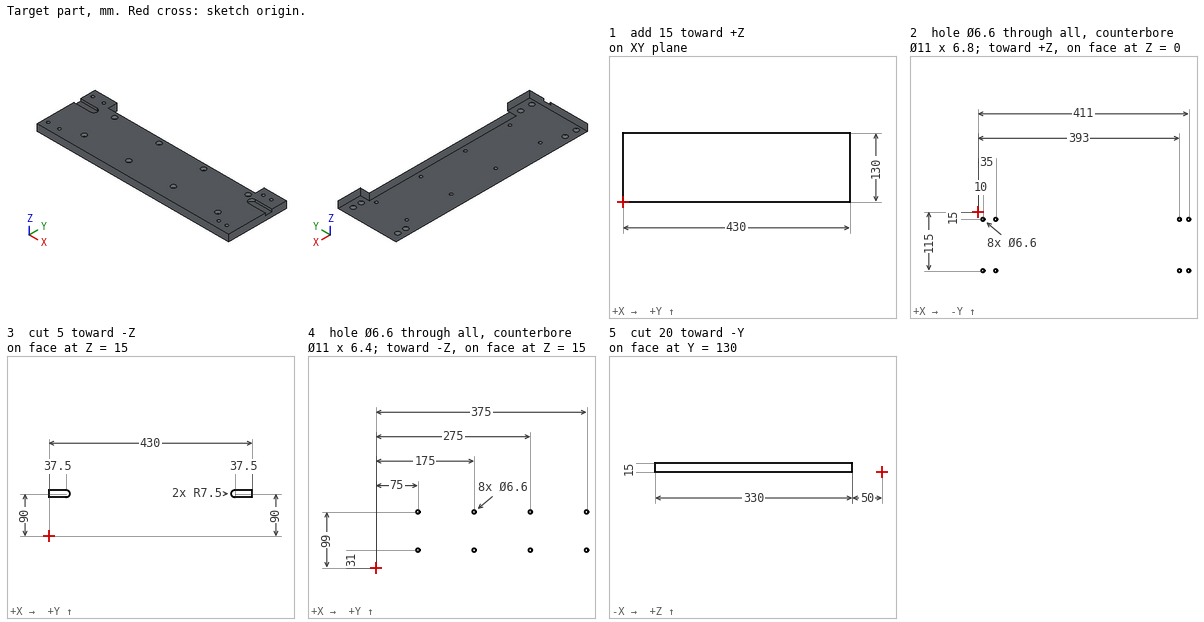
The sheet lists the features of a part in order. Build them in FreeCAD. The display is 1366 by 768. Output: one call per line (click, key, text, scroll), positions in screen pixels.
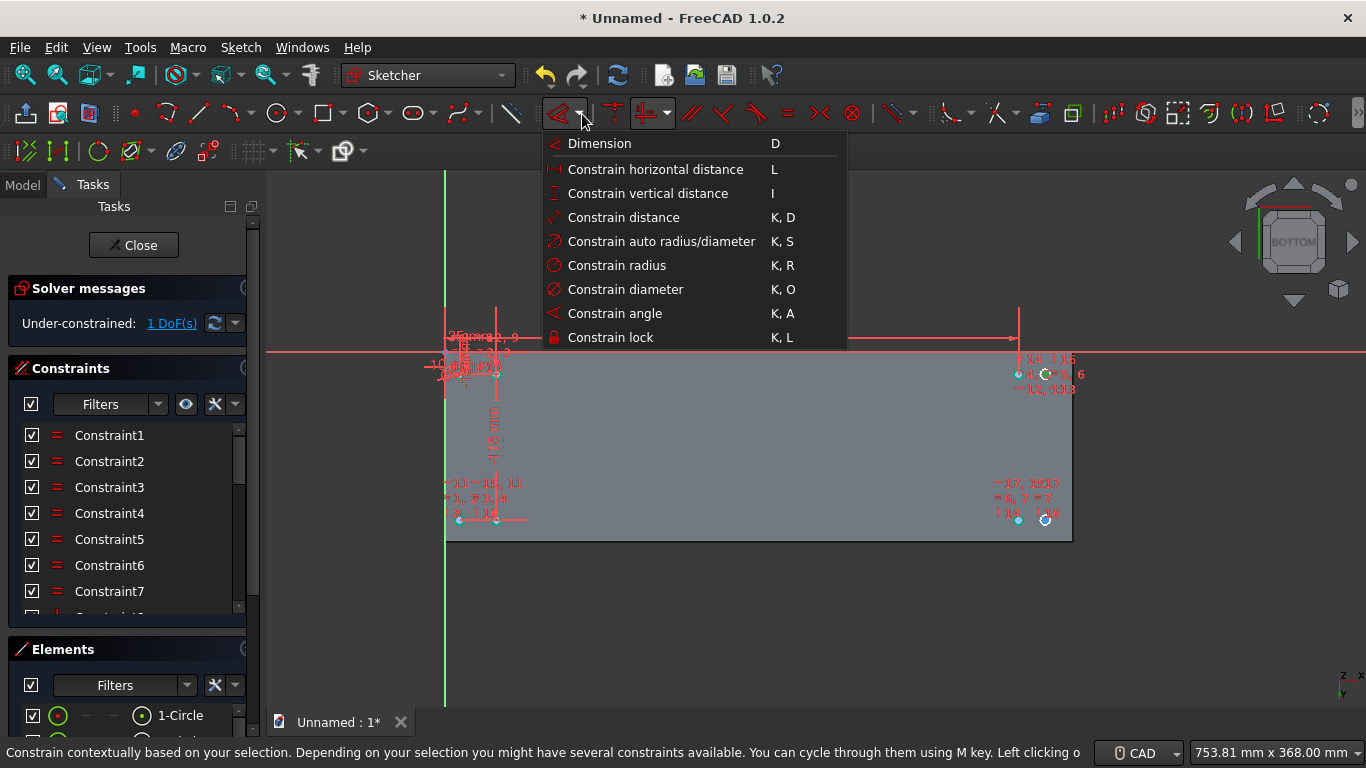
click(695, 169)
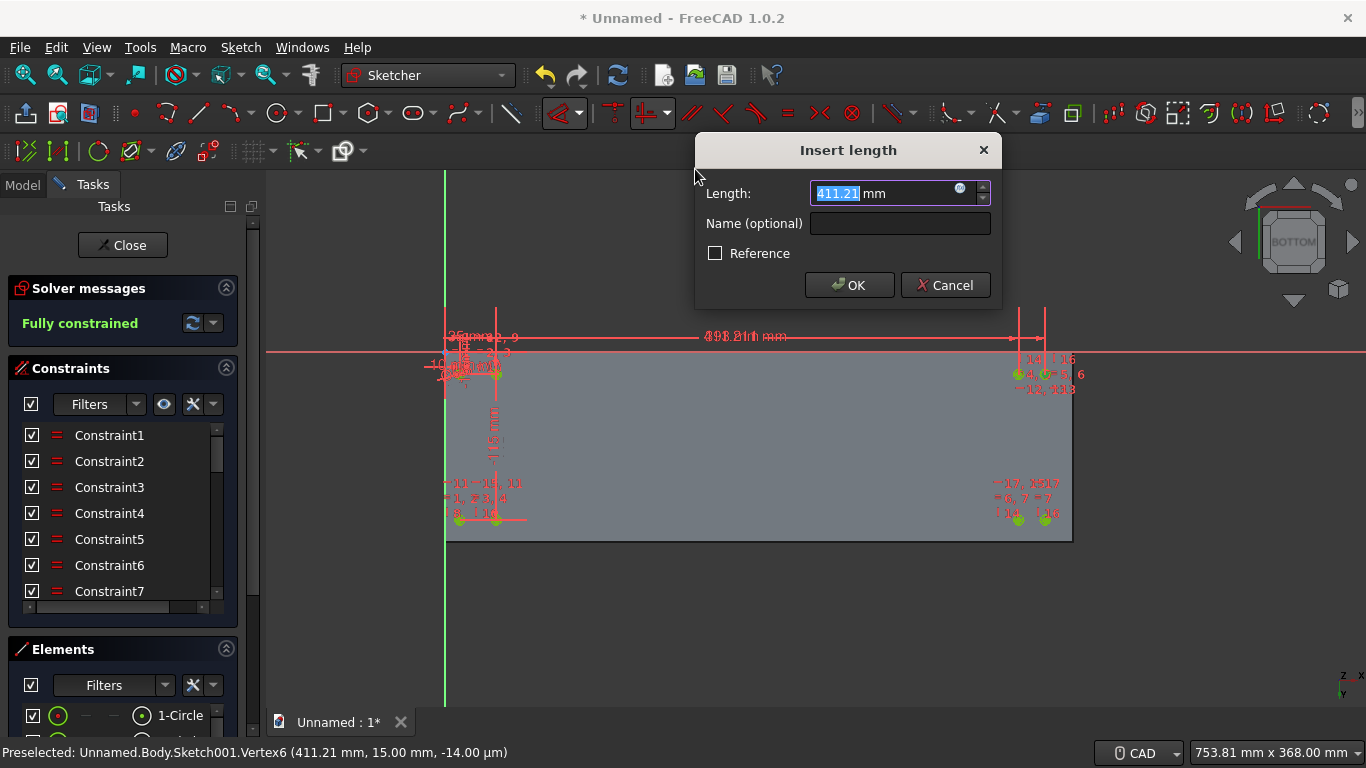
text(411)
key(Return)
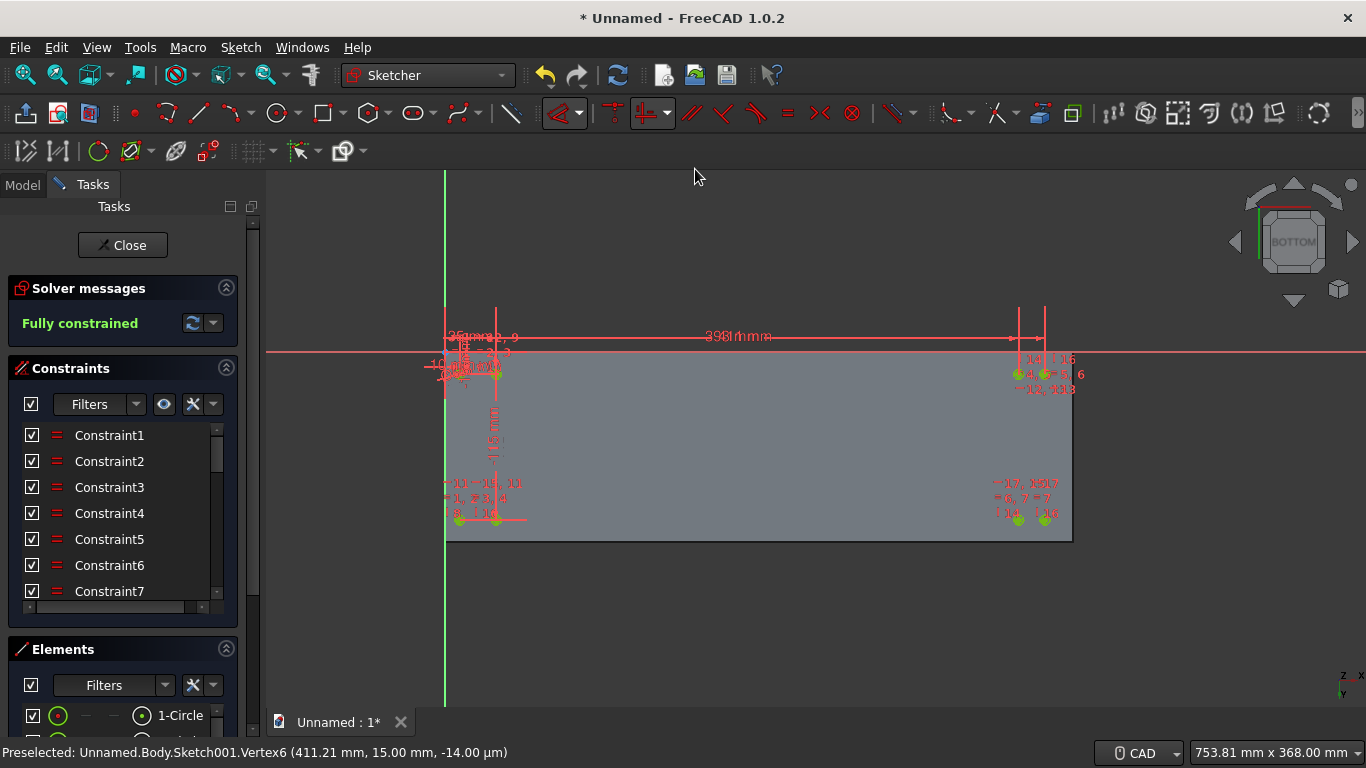
click(123, 245)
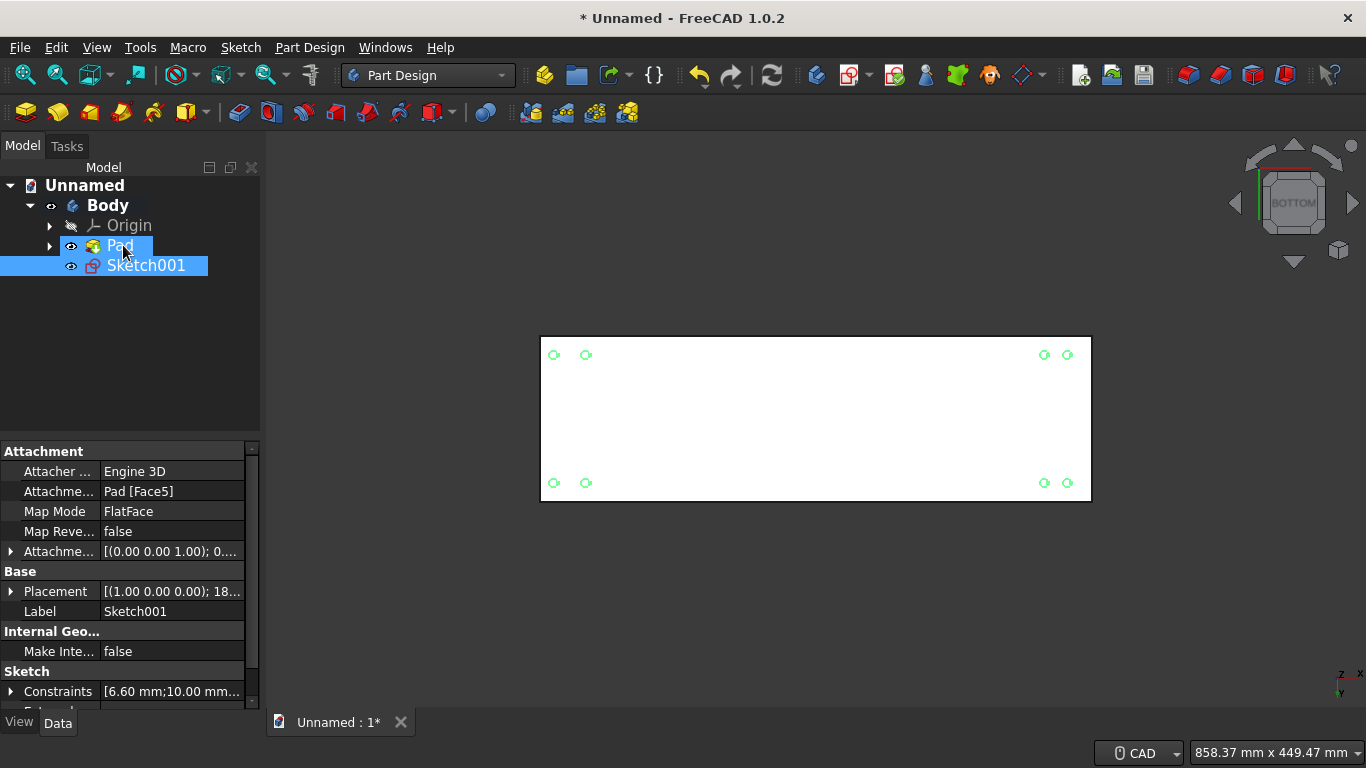
click(272, 112)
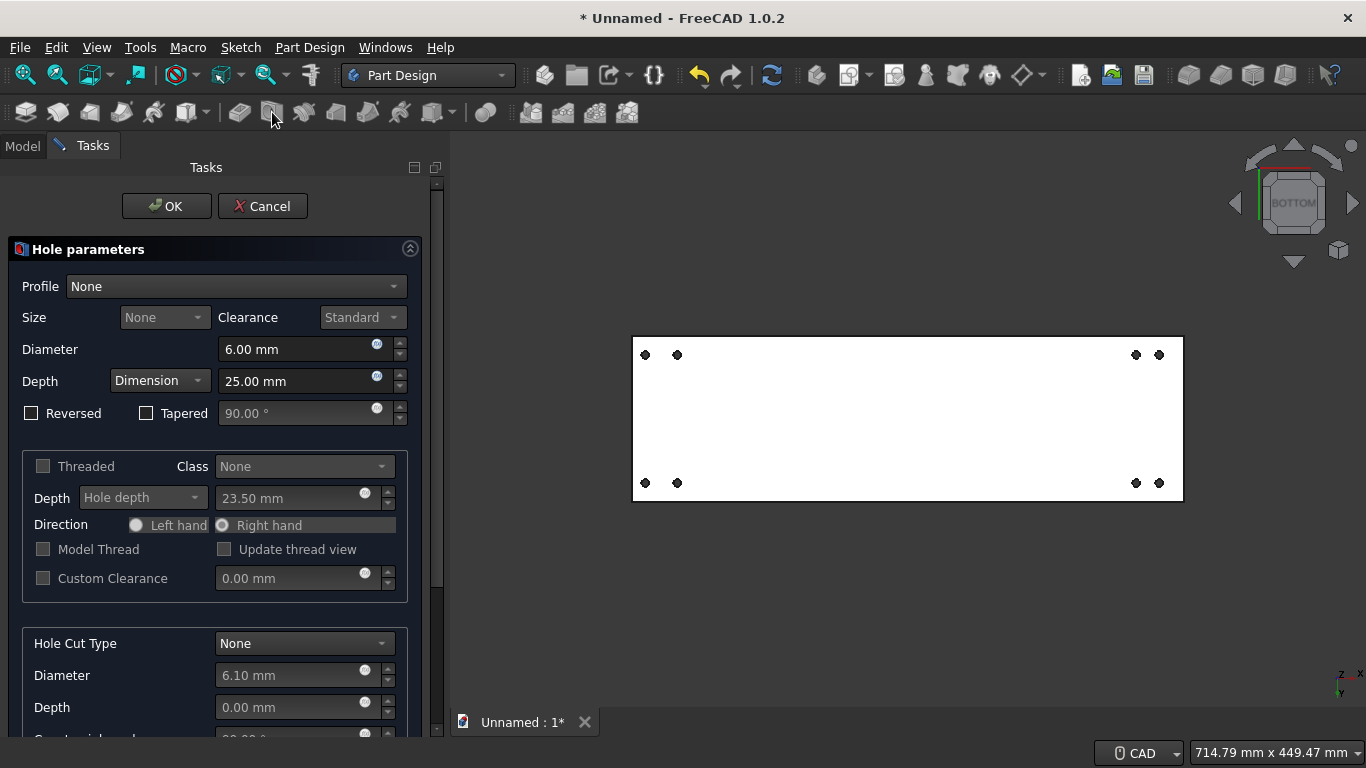
triple_click(305, 349)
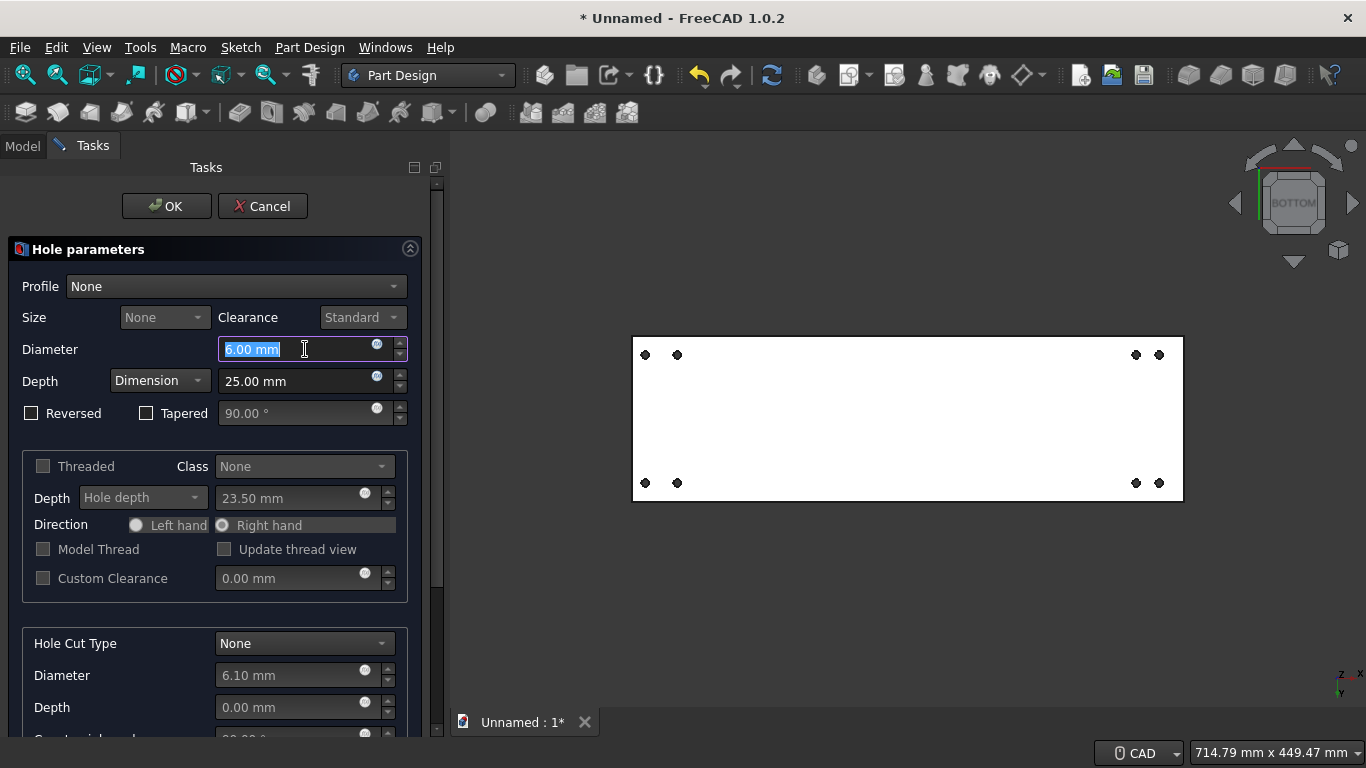
text(6.6)
key(Tab)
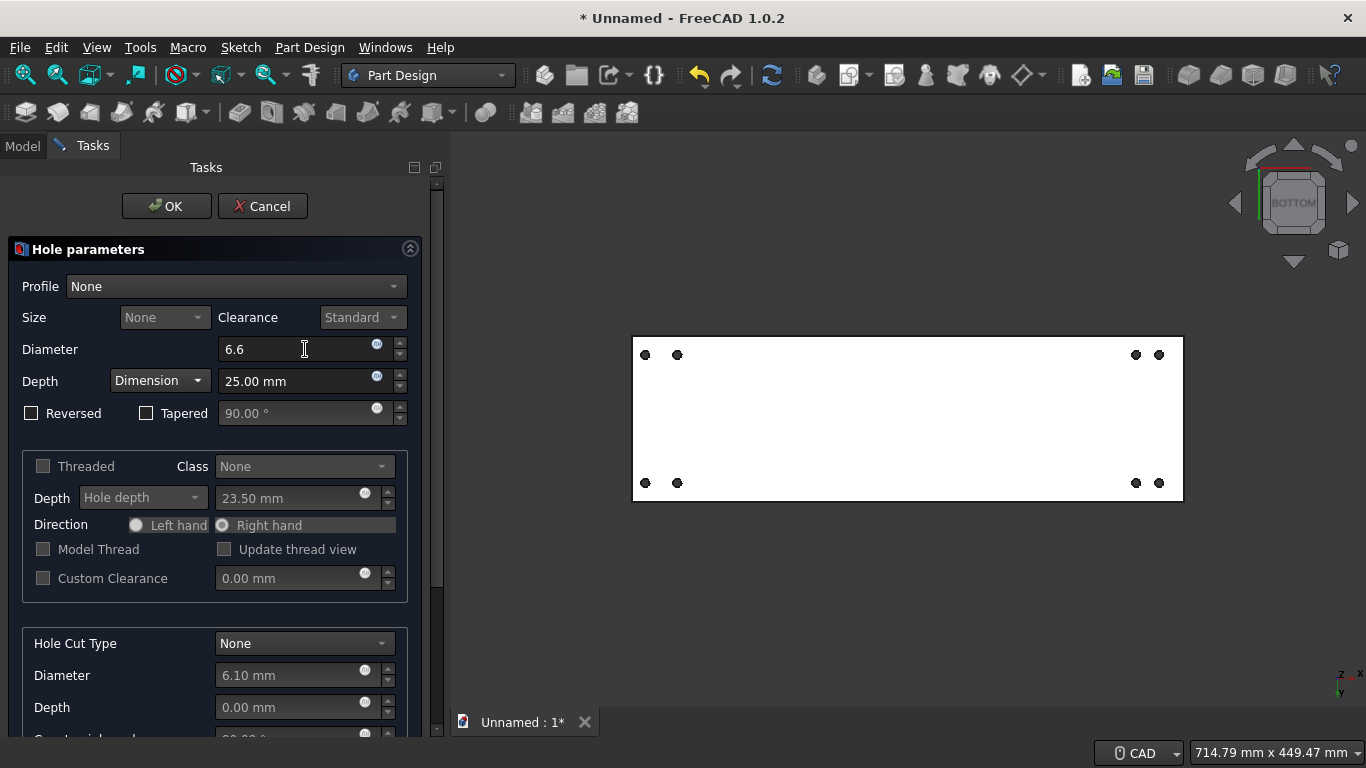
click(161, 380)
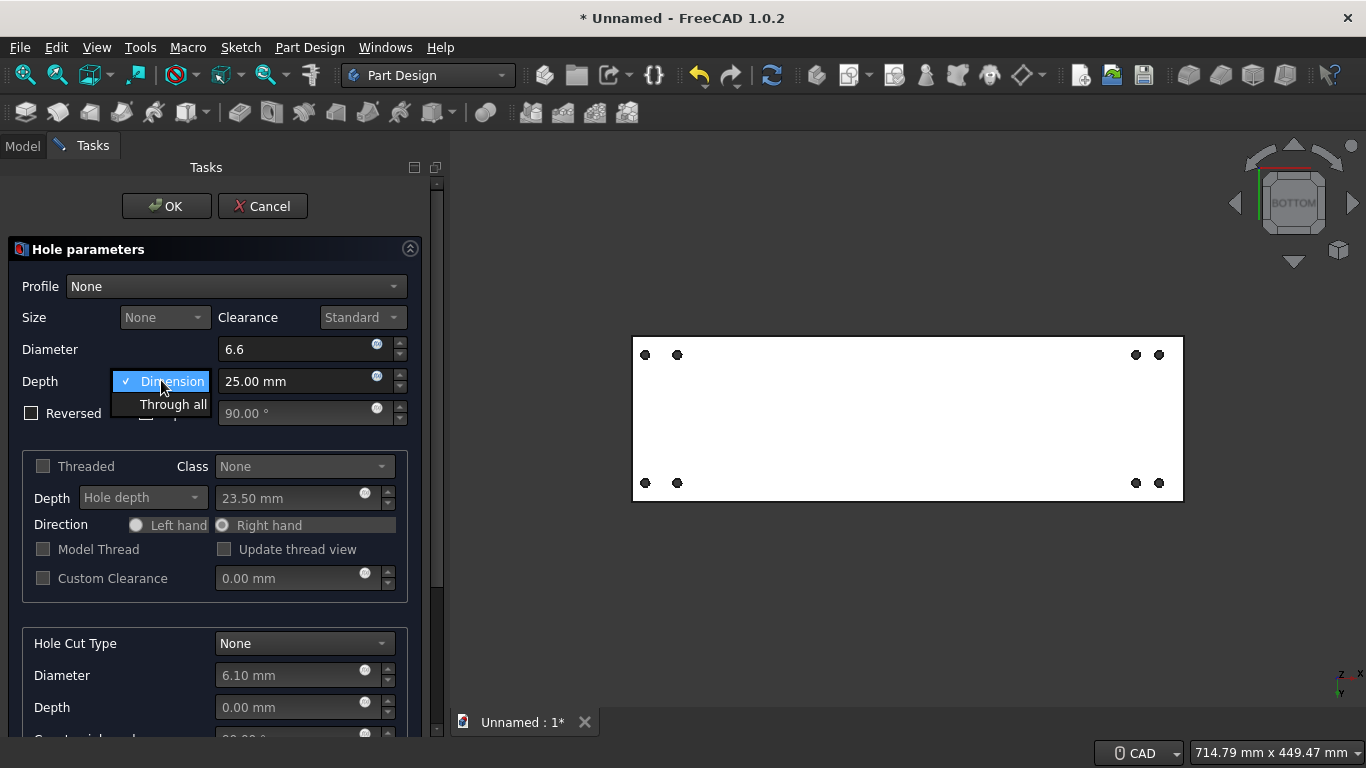
click(160, 404)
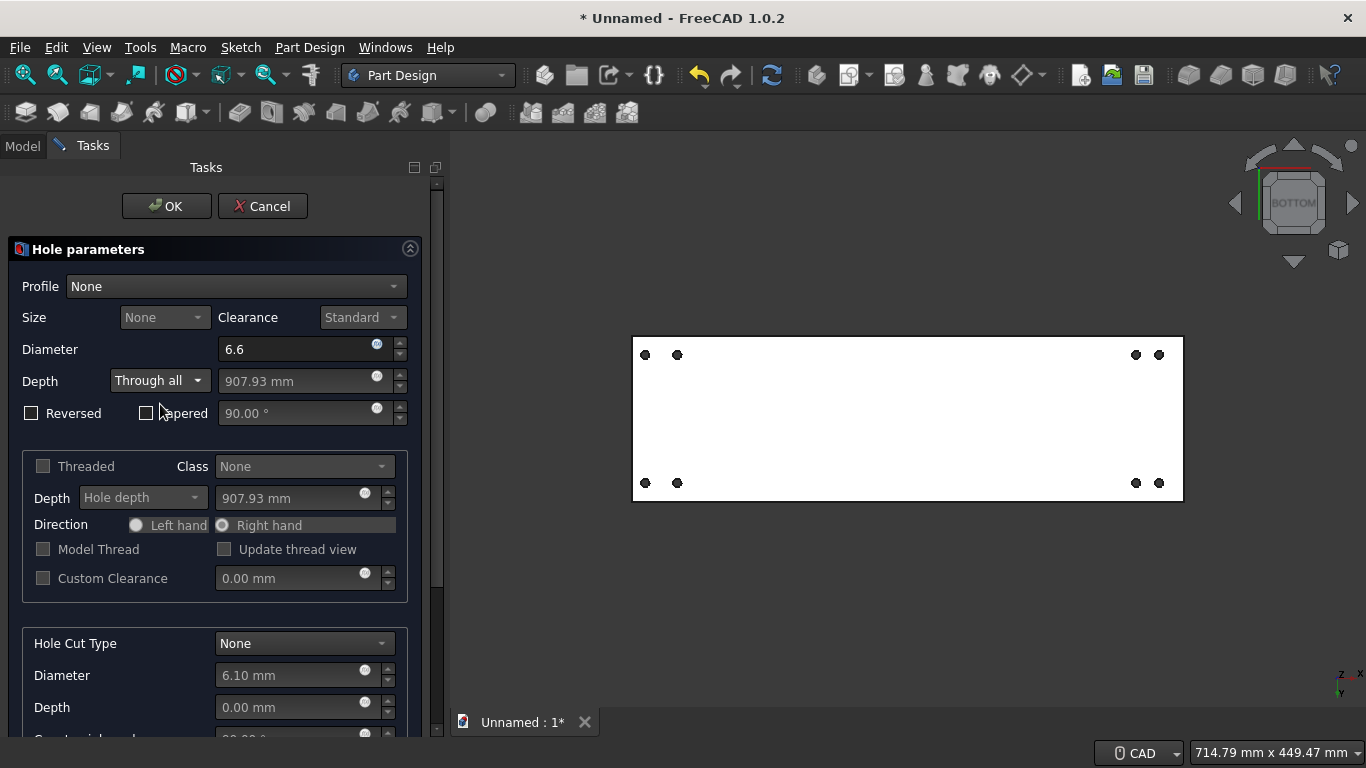
click(306, 644)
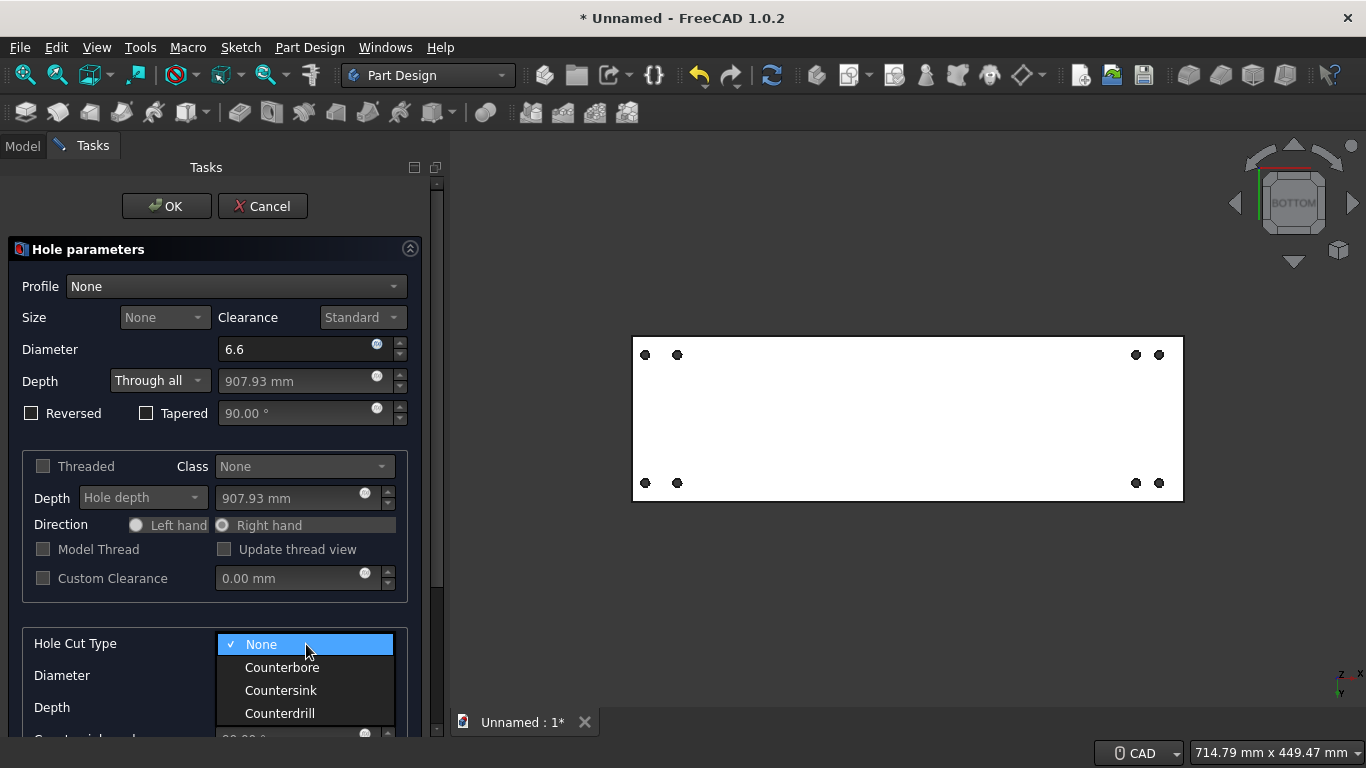
click(304, 668)